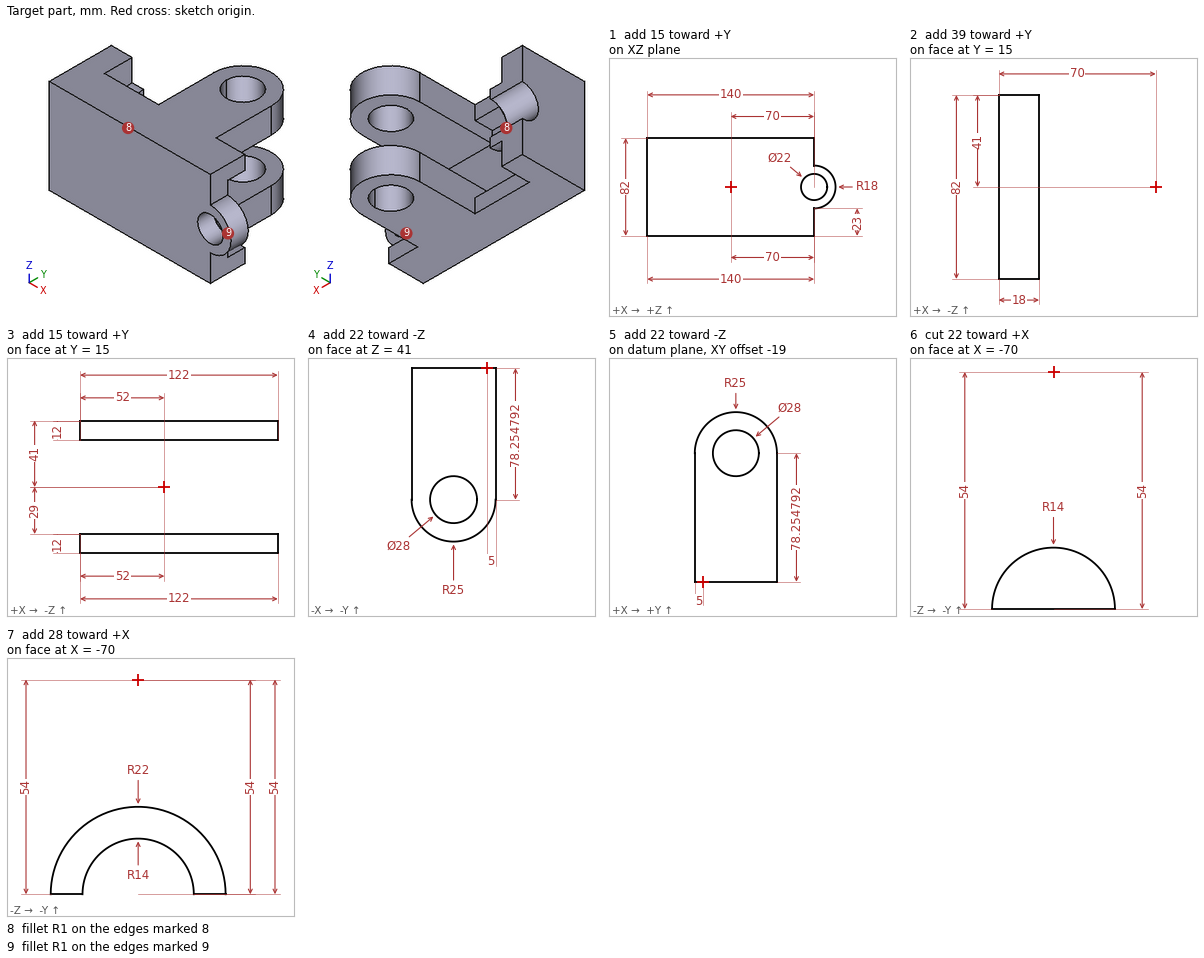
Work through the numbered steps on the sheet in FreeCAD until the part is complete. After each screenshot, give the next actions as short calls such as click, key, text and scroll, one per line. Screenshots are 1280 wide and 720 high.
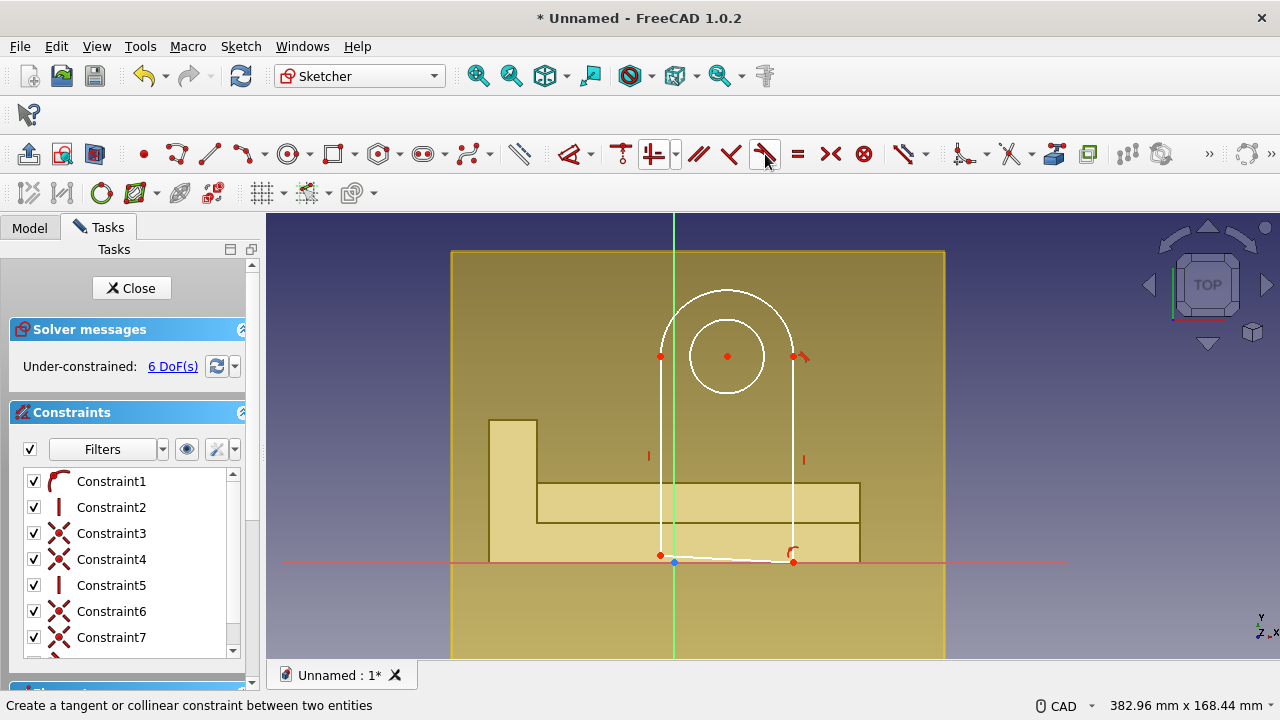
click(661, 496)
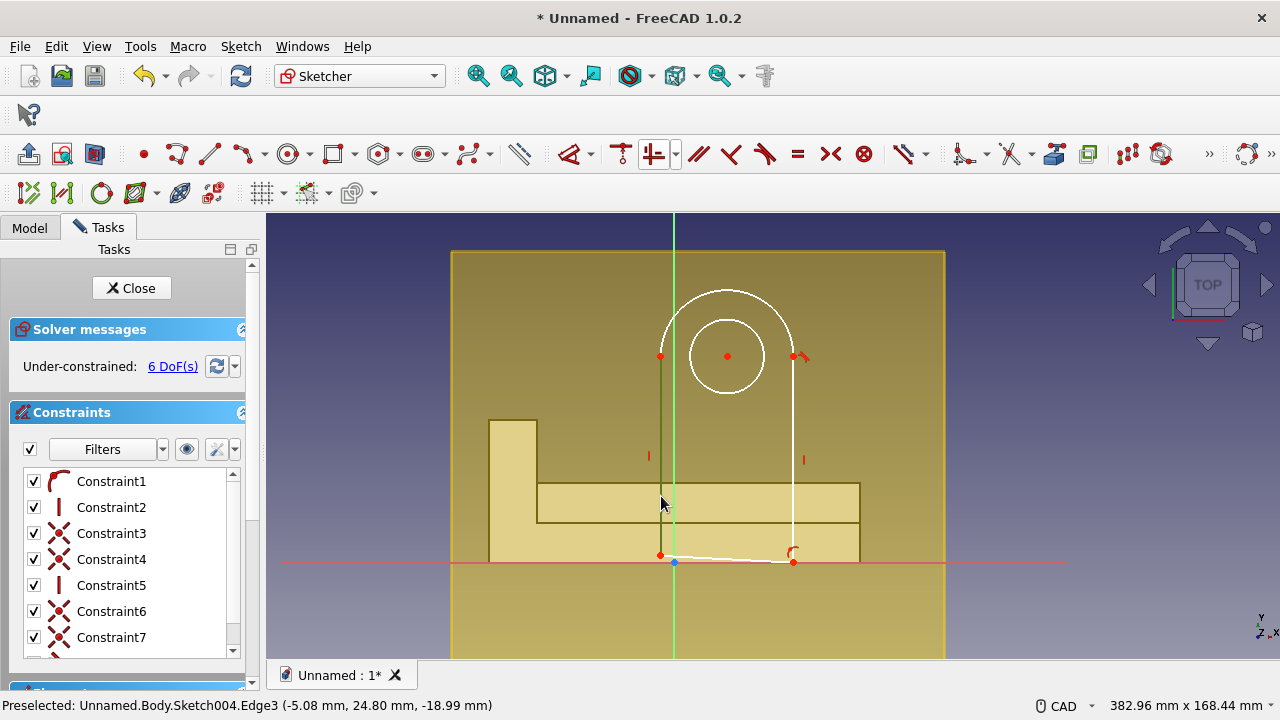
click(766, 303)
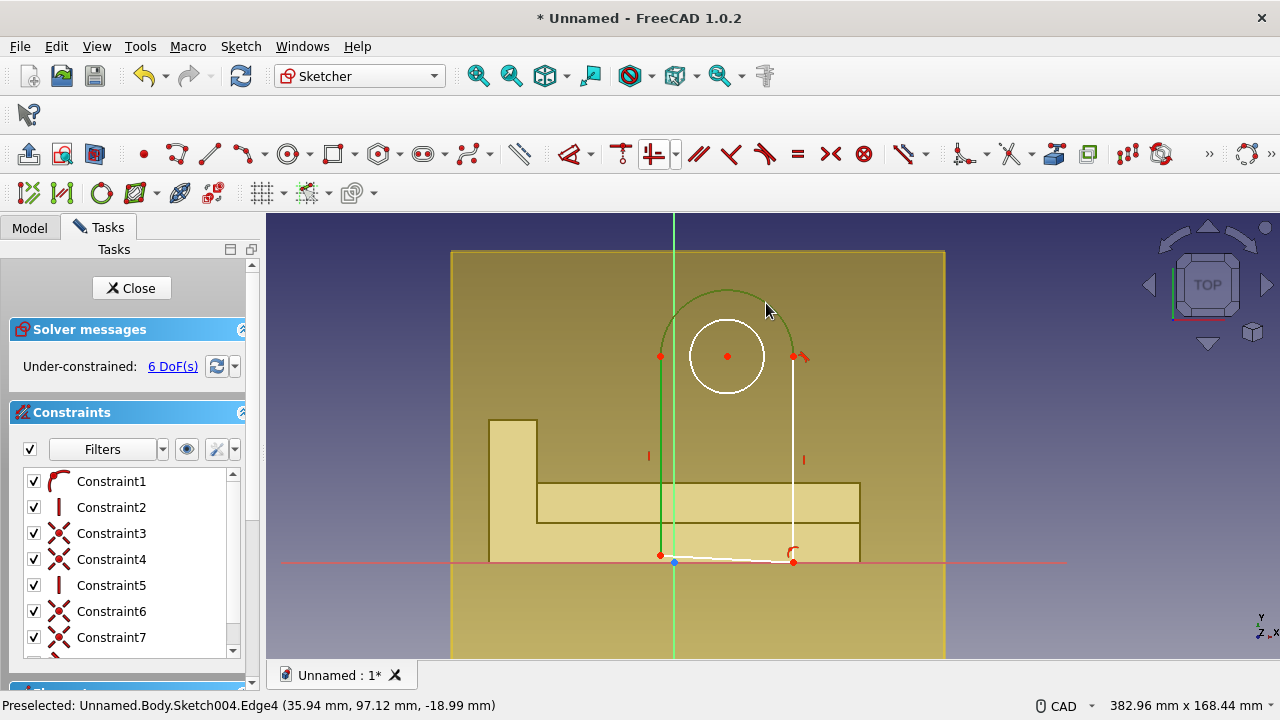
click(765, 154)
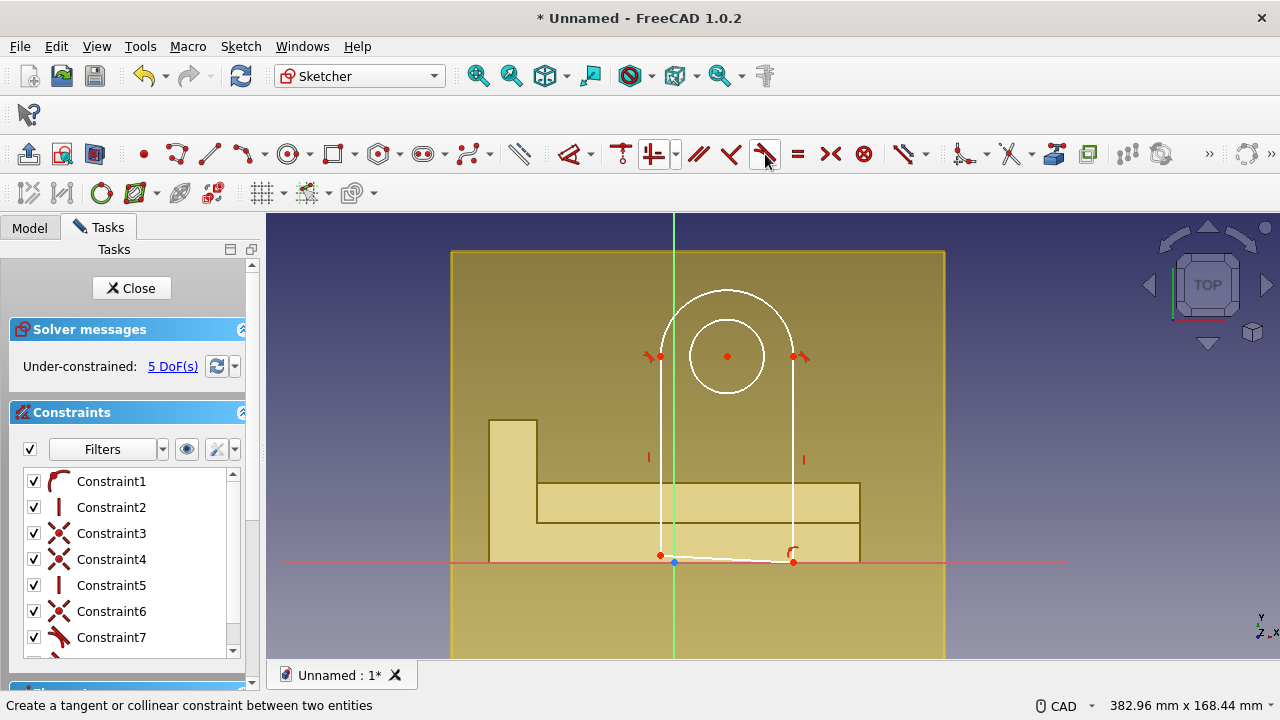
click(754, 561)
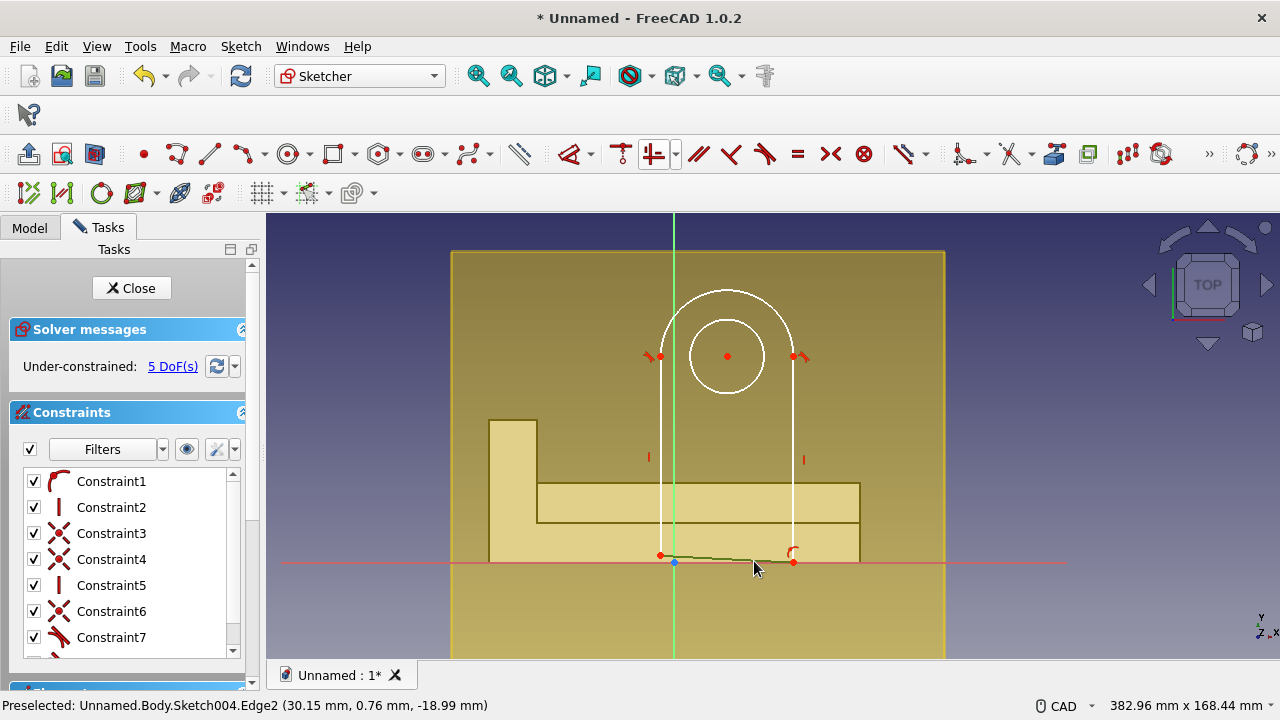
click(676, 154)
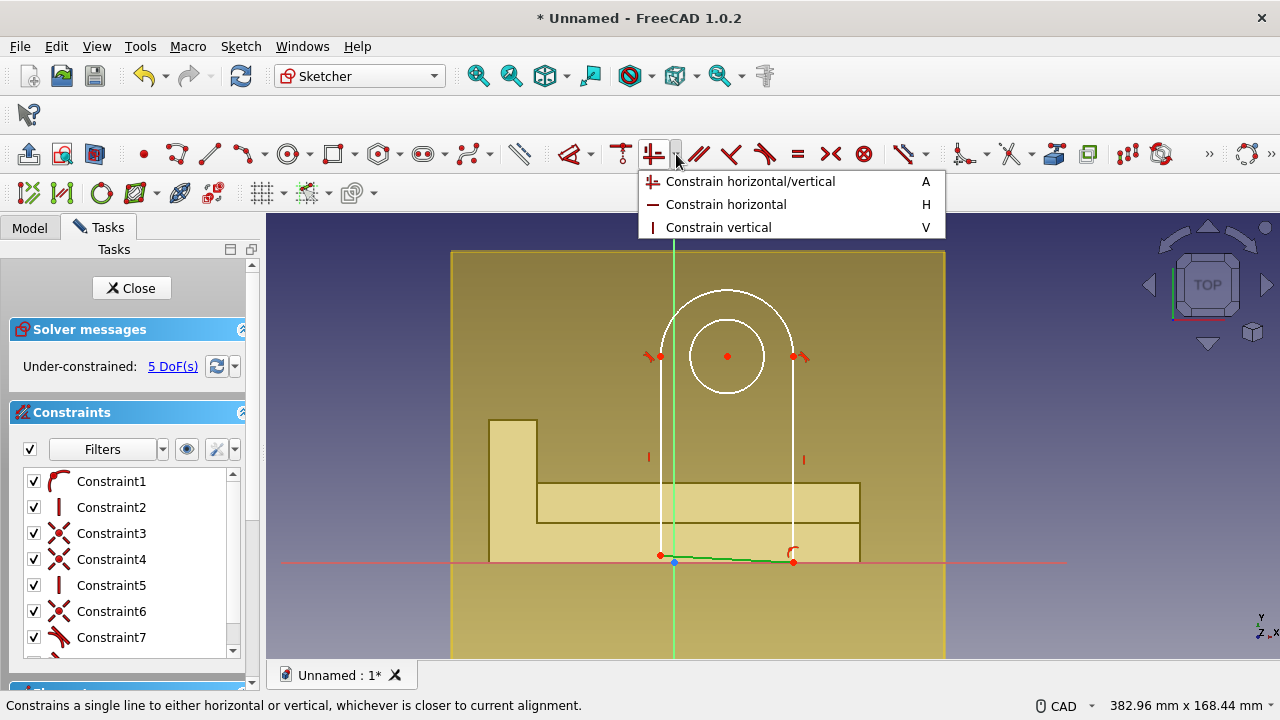
click(792, 204)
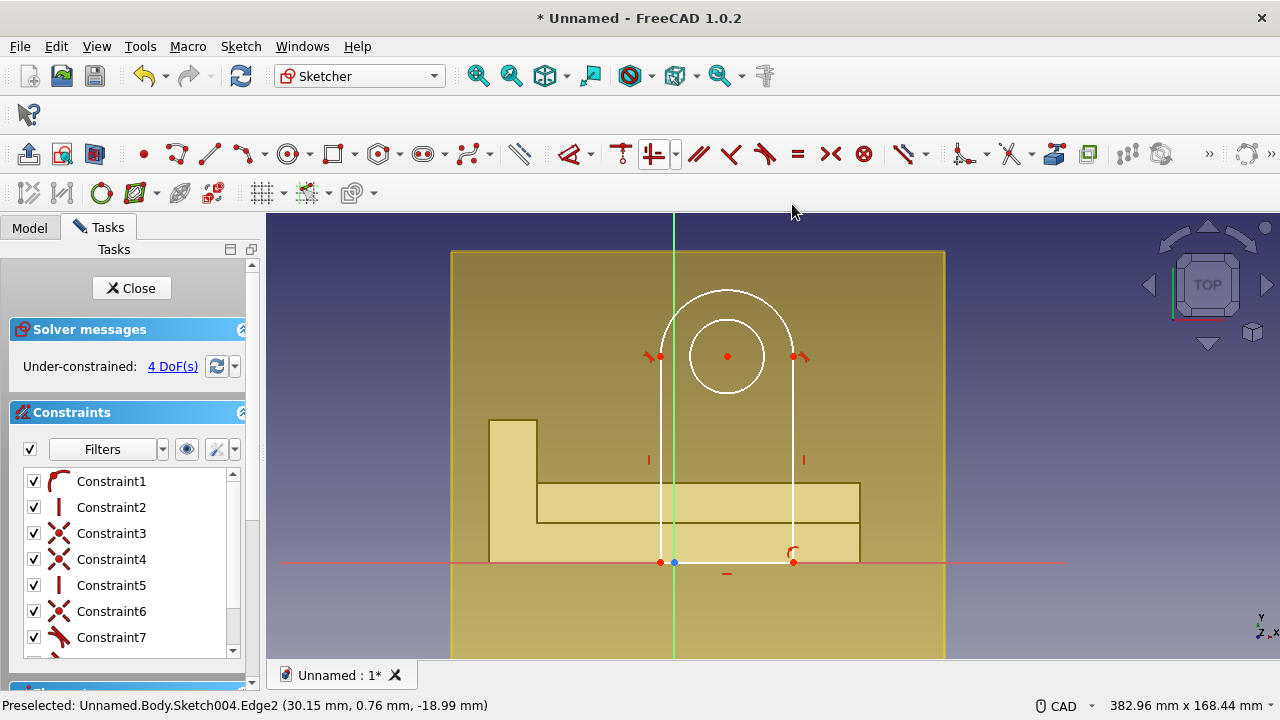
click(568, 154)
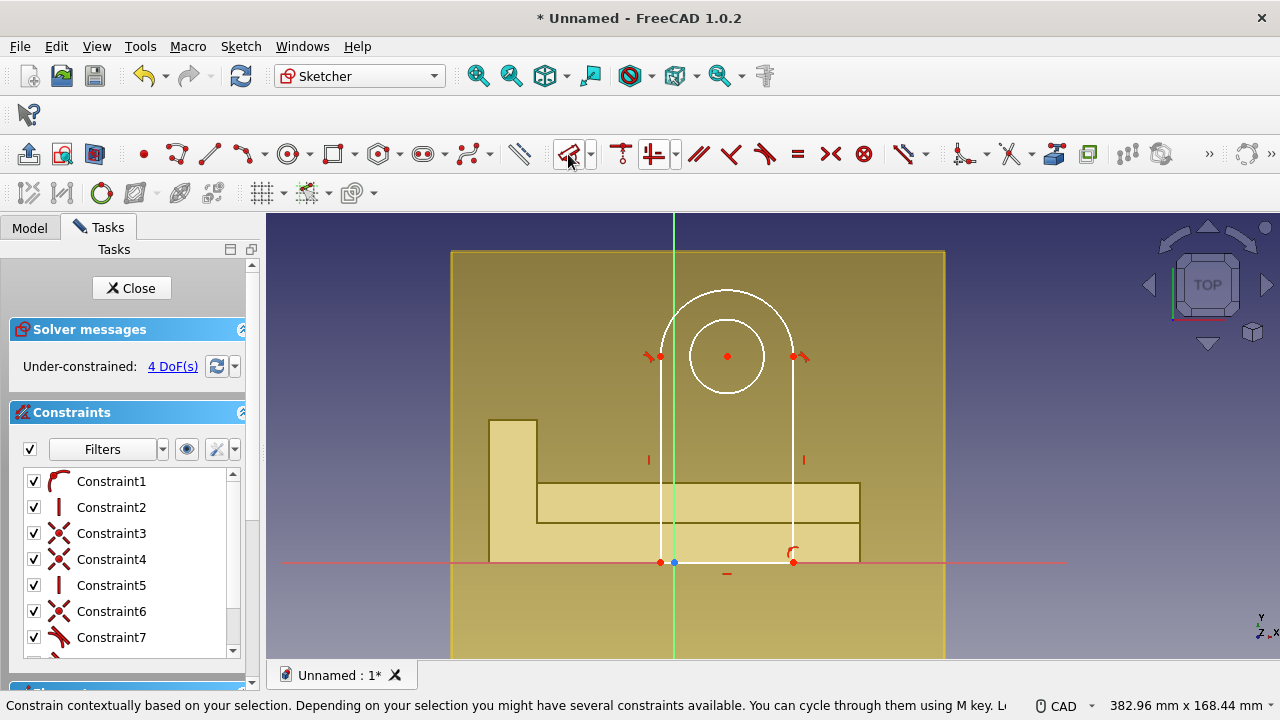
click(766, 303)
click(785, 277)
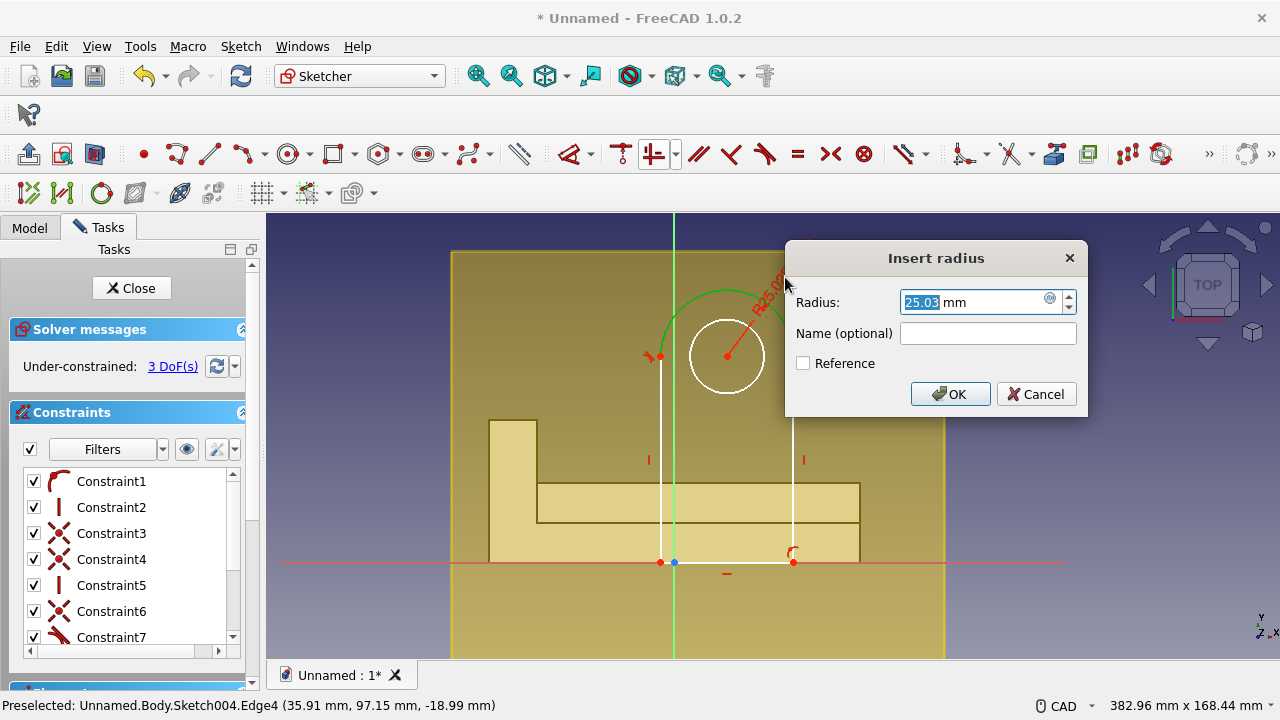
text(25)
key(Return)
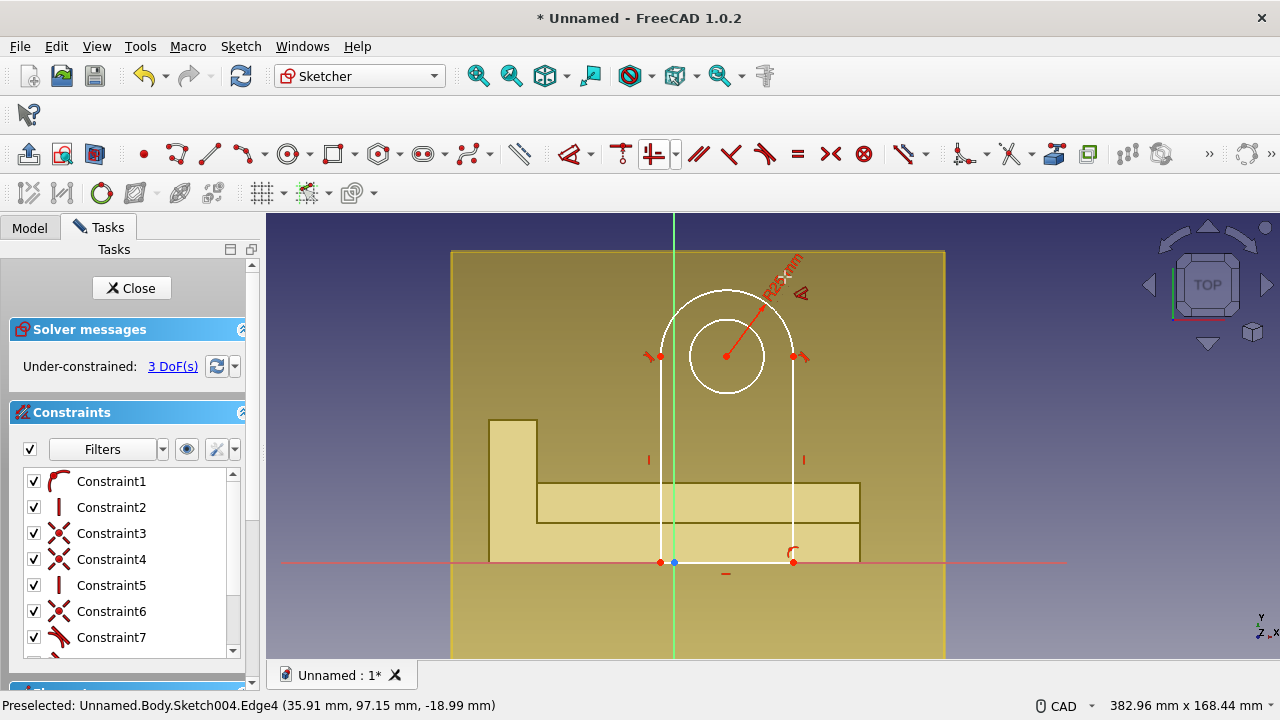
click(753, 330)
click(776, 405)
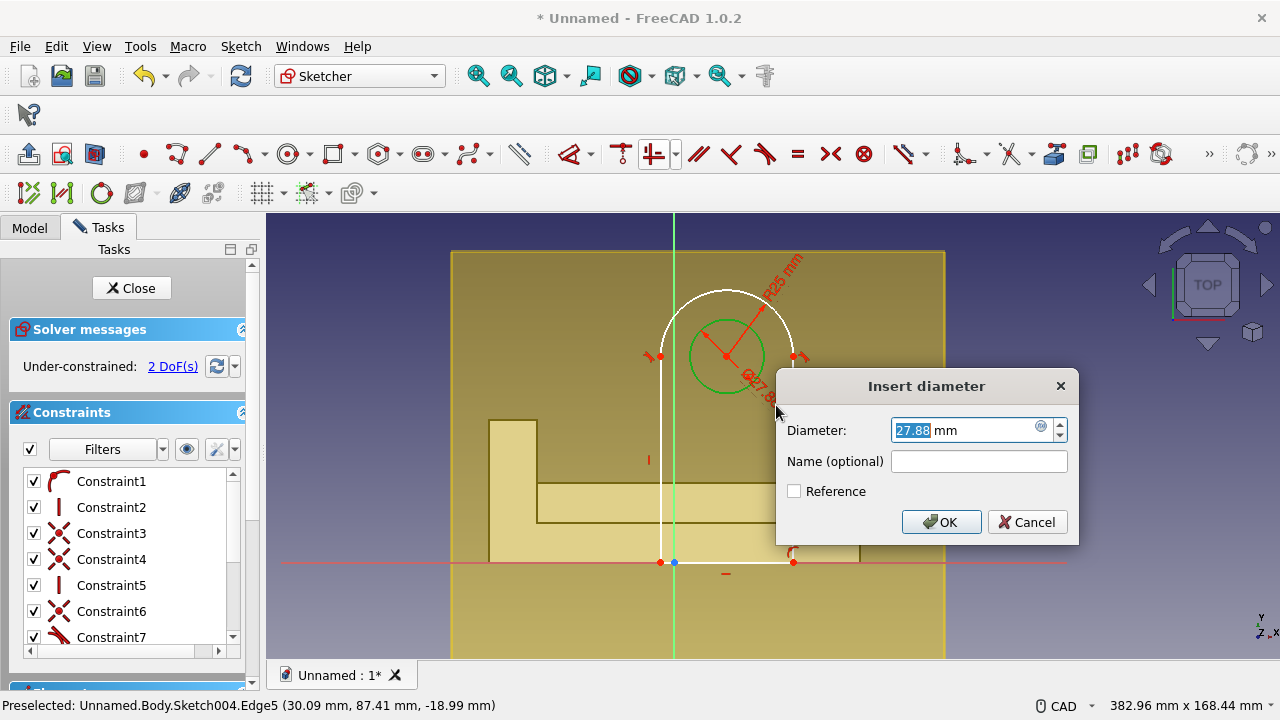
text(28)
key(Return)